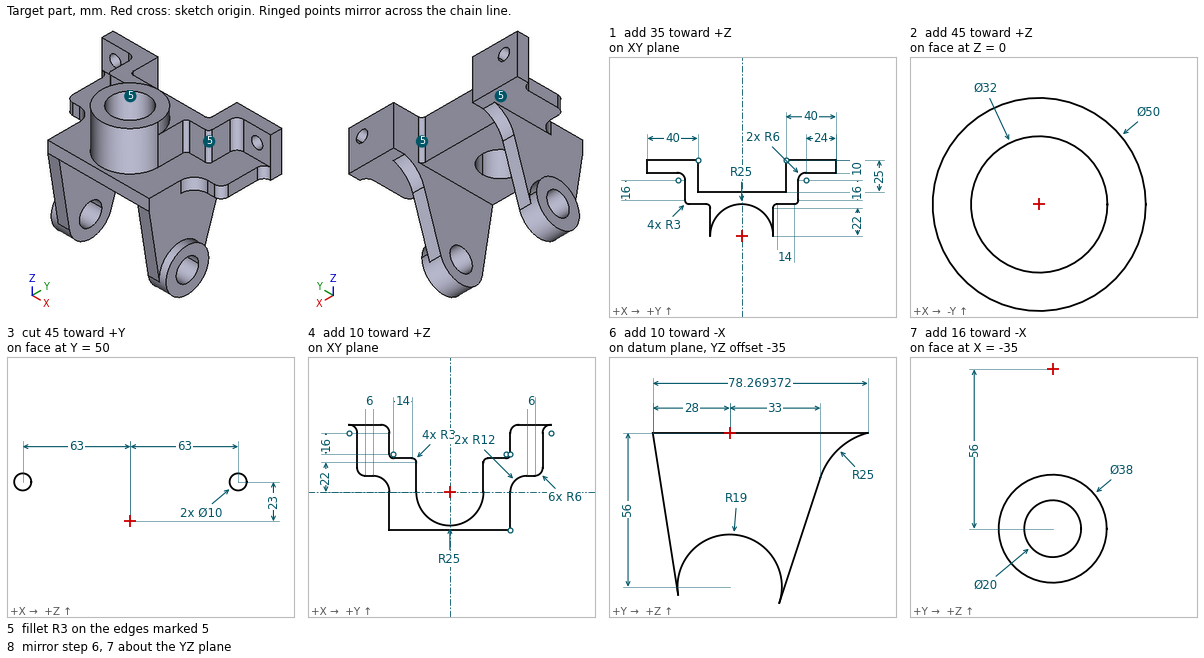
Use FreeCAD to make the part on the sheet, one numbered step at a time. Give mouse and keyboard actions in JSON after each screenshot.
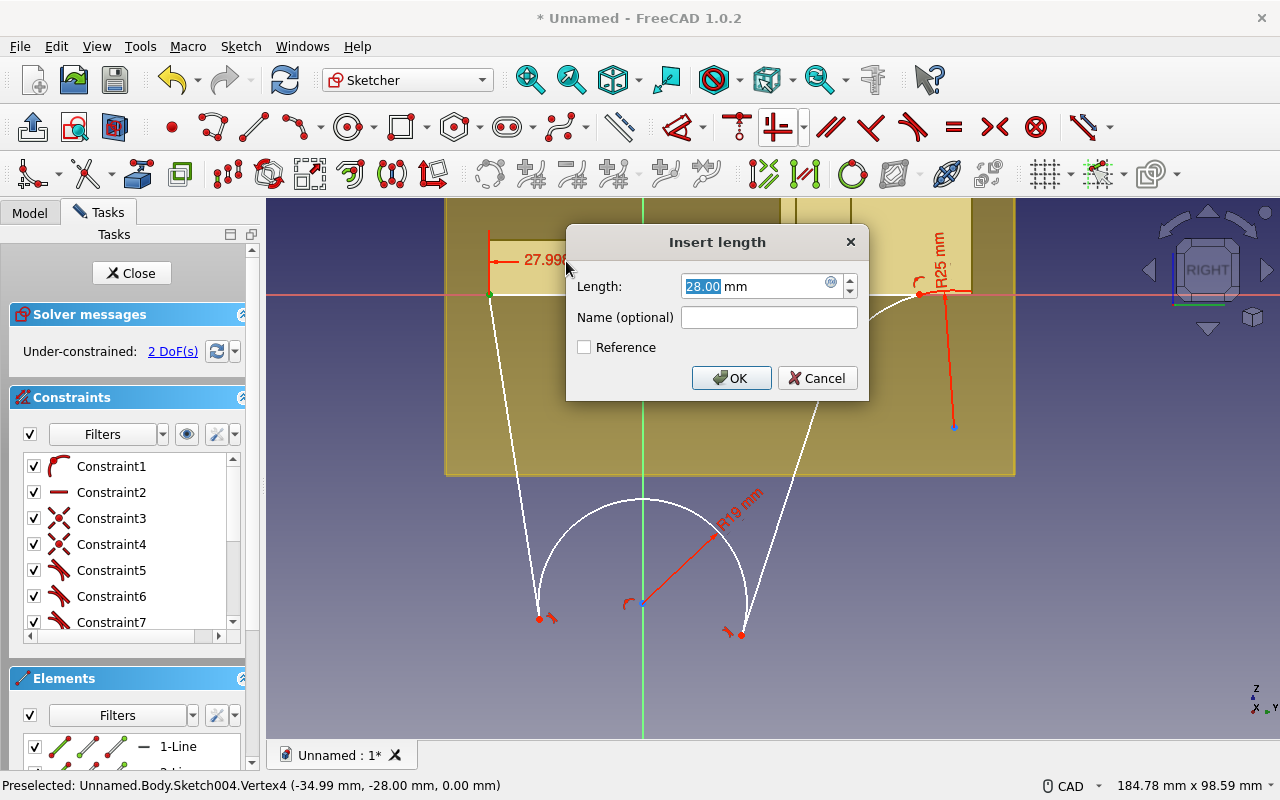
{"action": "type", "text": "28"}
{"action": "key", "text": "Return"}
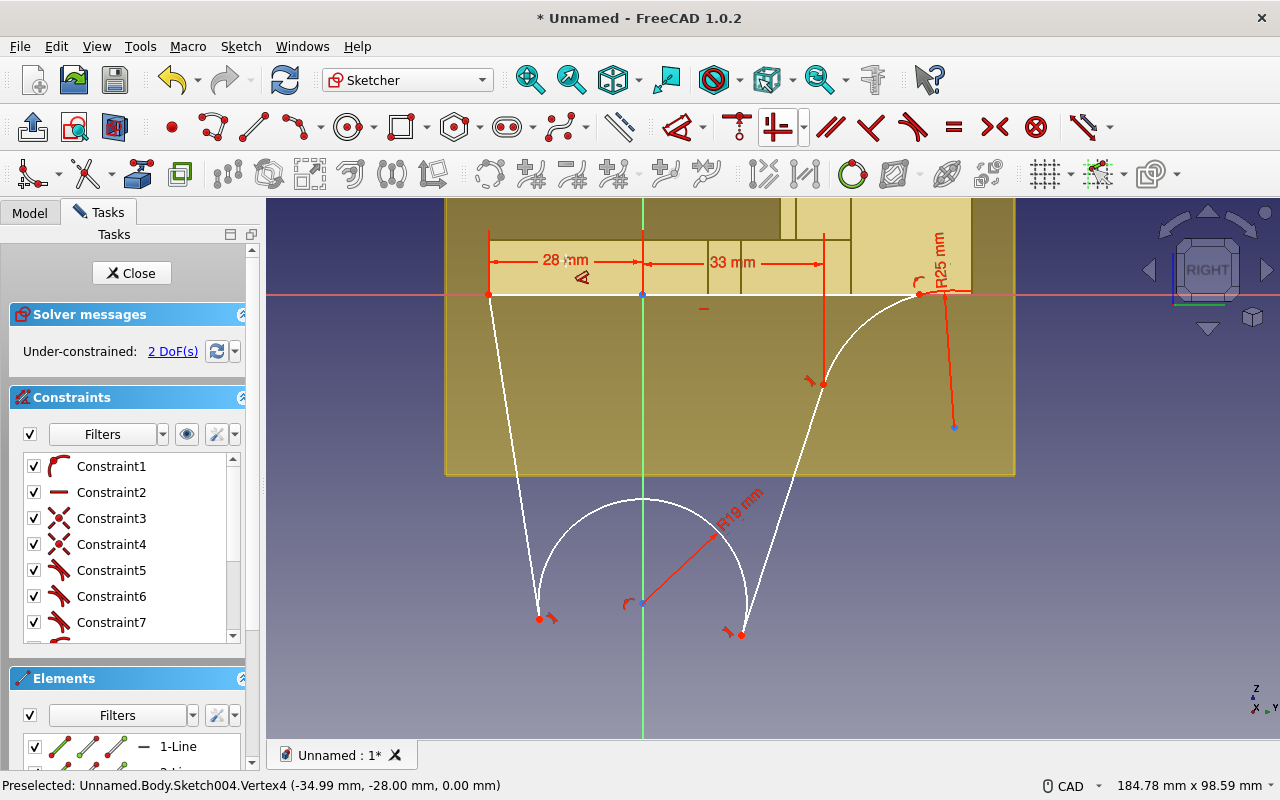
{"action": "left_click", "coordinate": [643, 603]}
{"action": "left_click", "coordinate": [609, 449]}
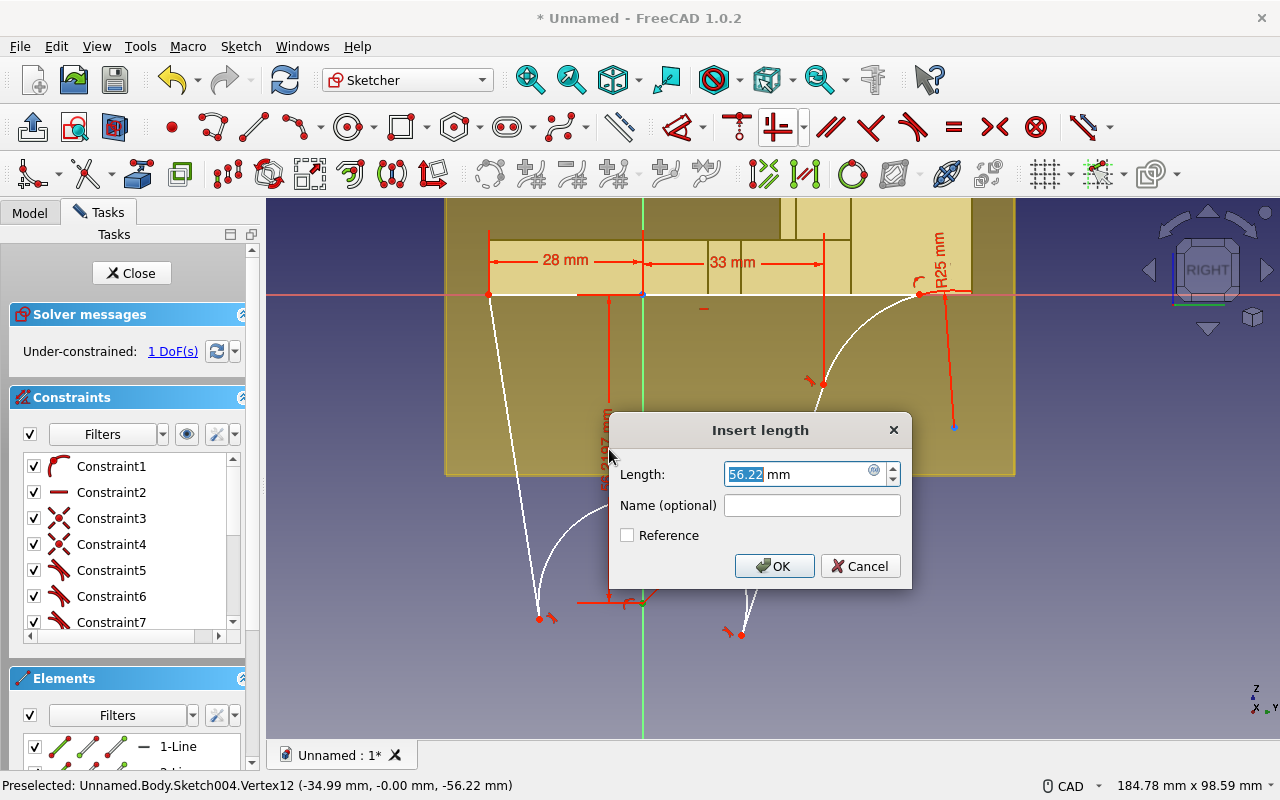
{"action": "type", "text": "56"}
{"action": "key", "text": "Return"}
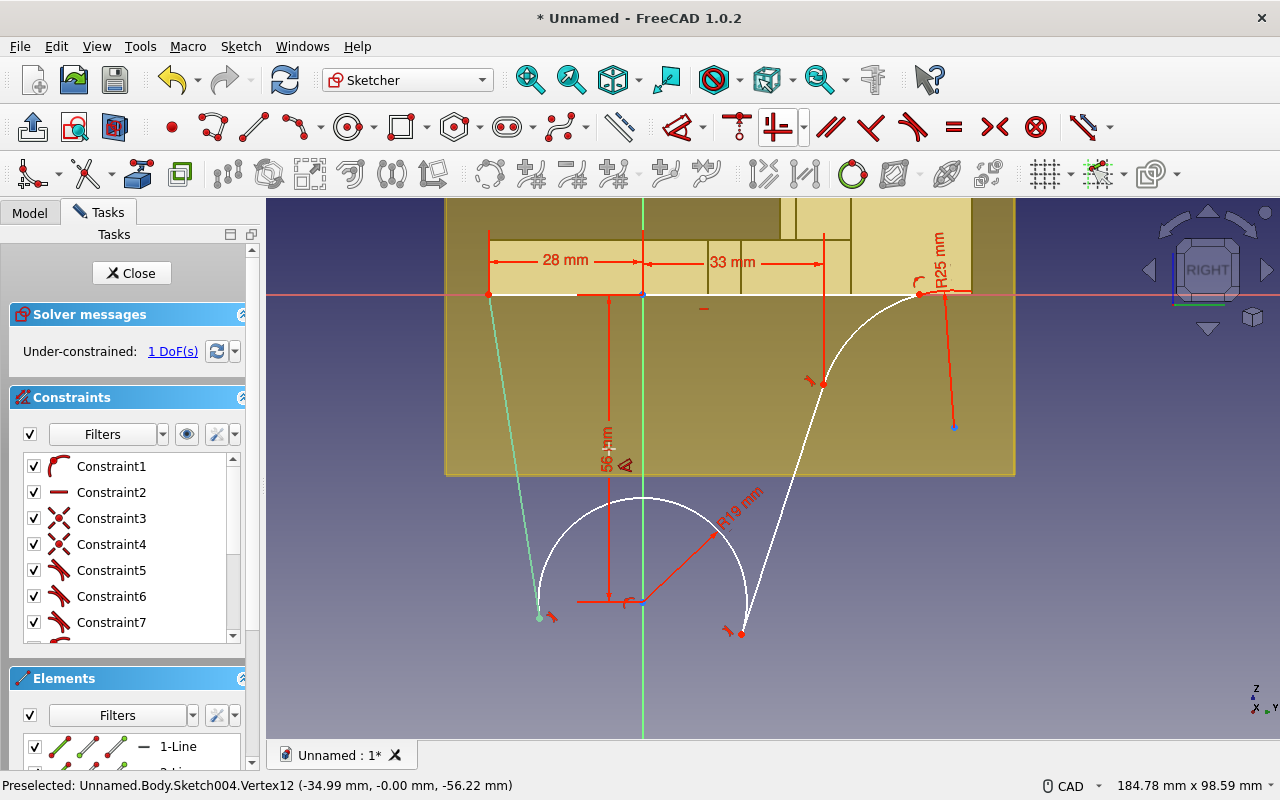
{"action": "left_click", "coordinate": [790, 295]}
{"action": "left_click", "coordinate": [855, 261]}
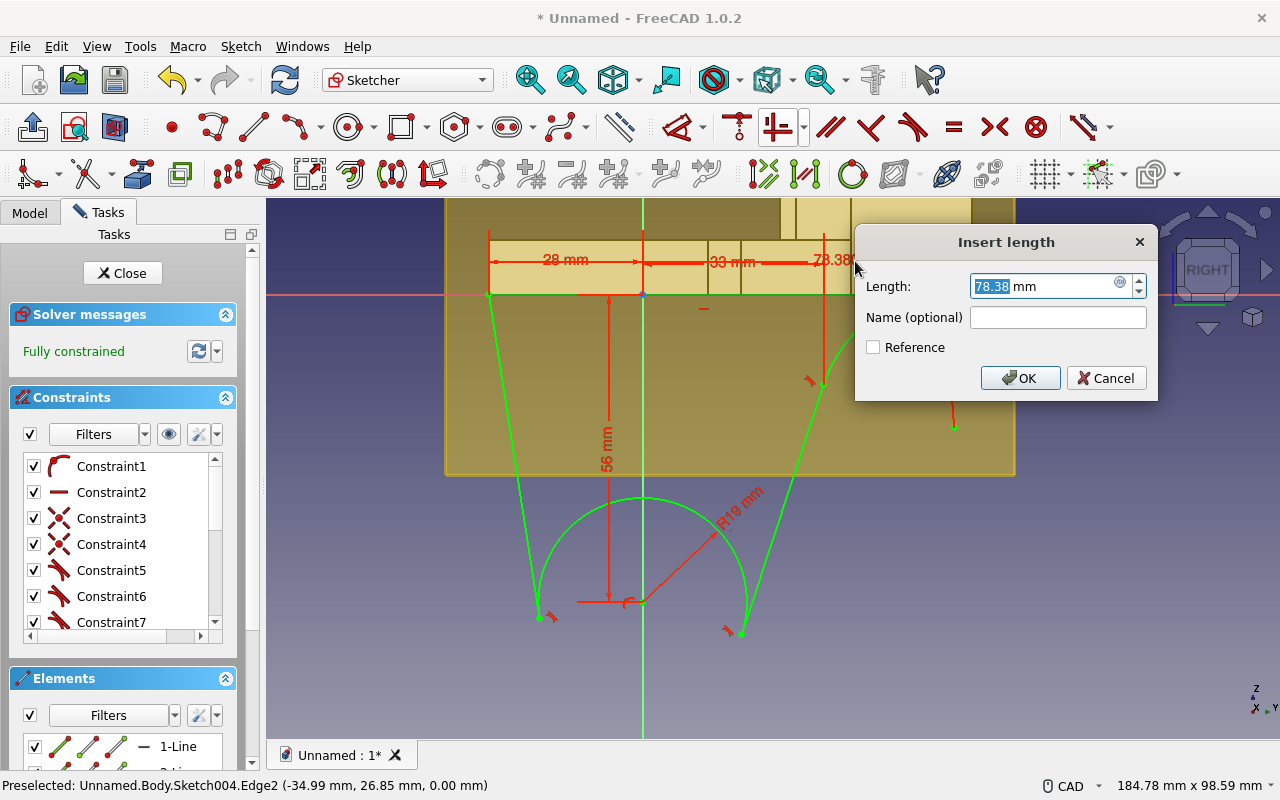
{"action": "type", "text": "78.269372"}
{"action": "key", "text": "Return"}
{"action": "key", "text": "Escape"}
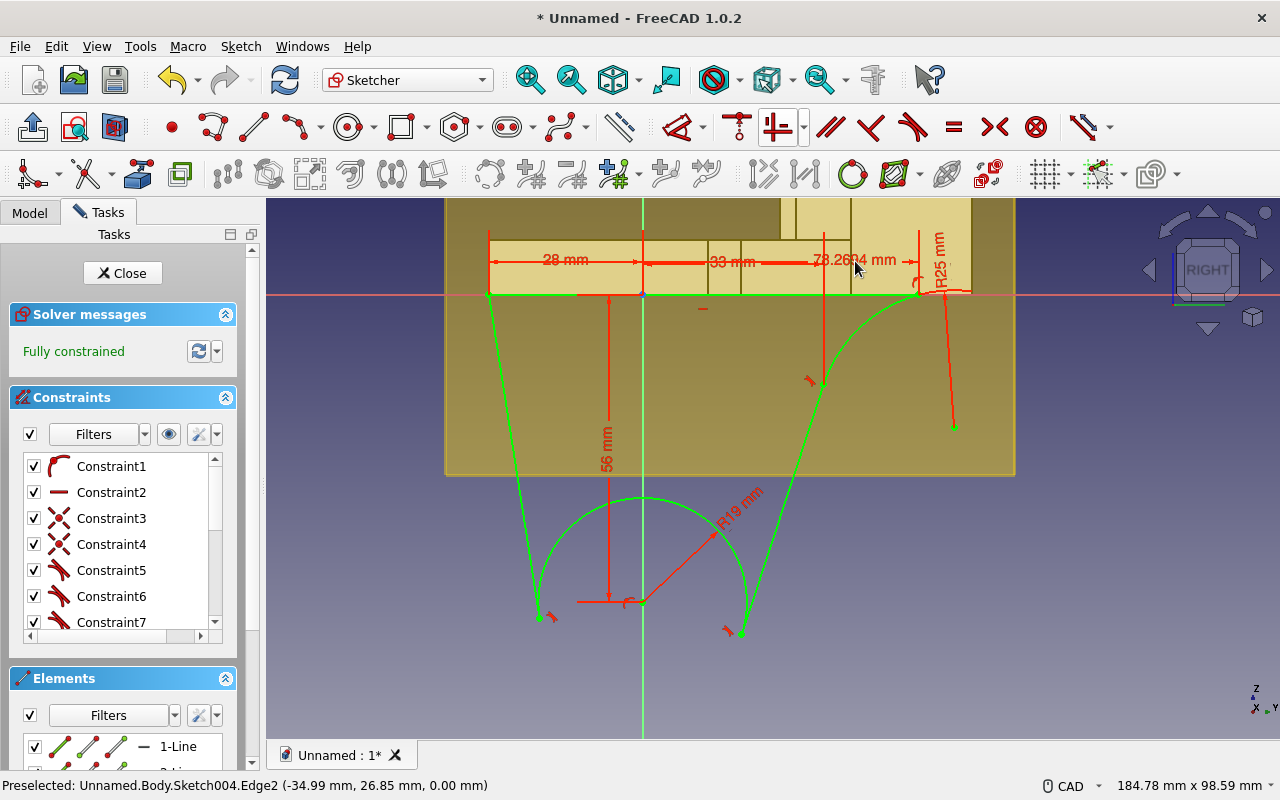
{"action": "left_click", "coordinate": [123, 273]}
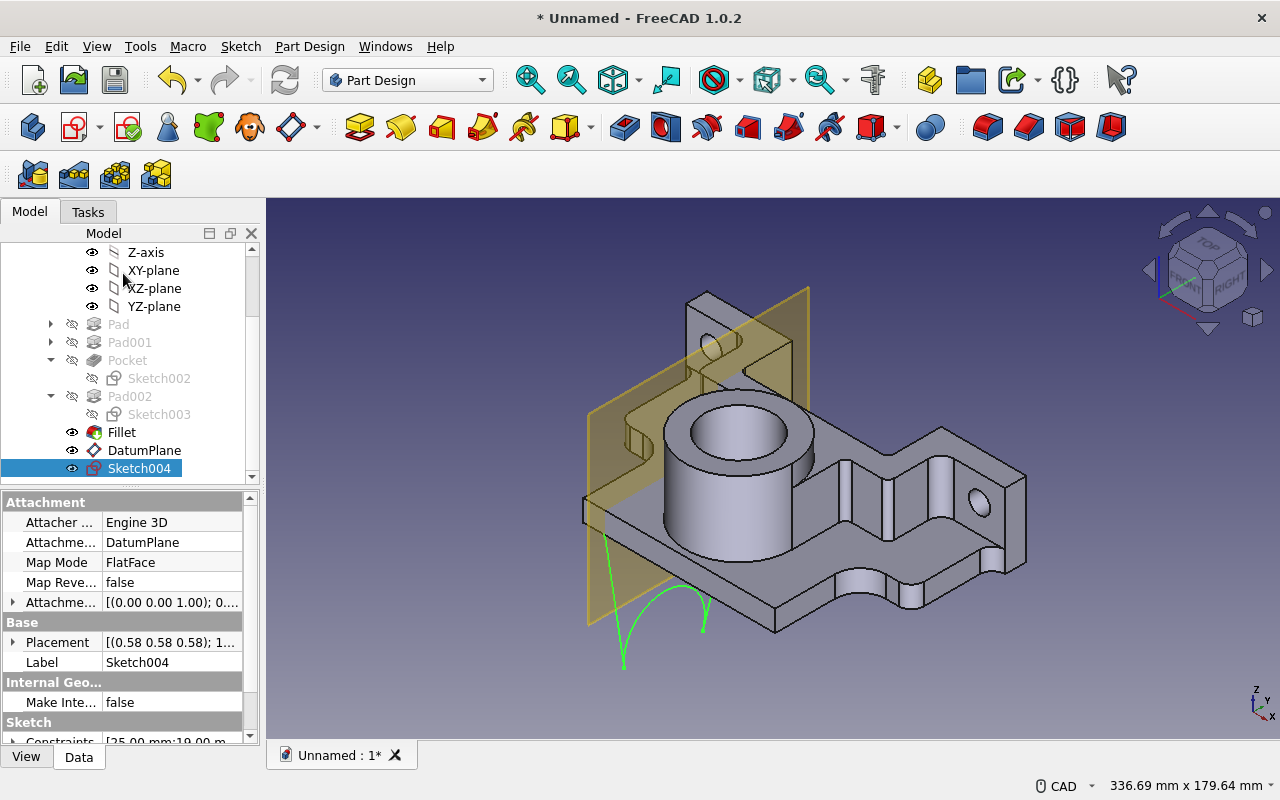
{"action": "left_click", "coordinate": [360, 128]}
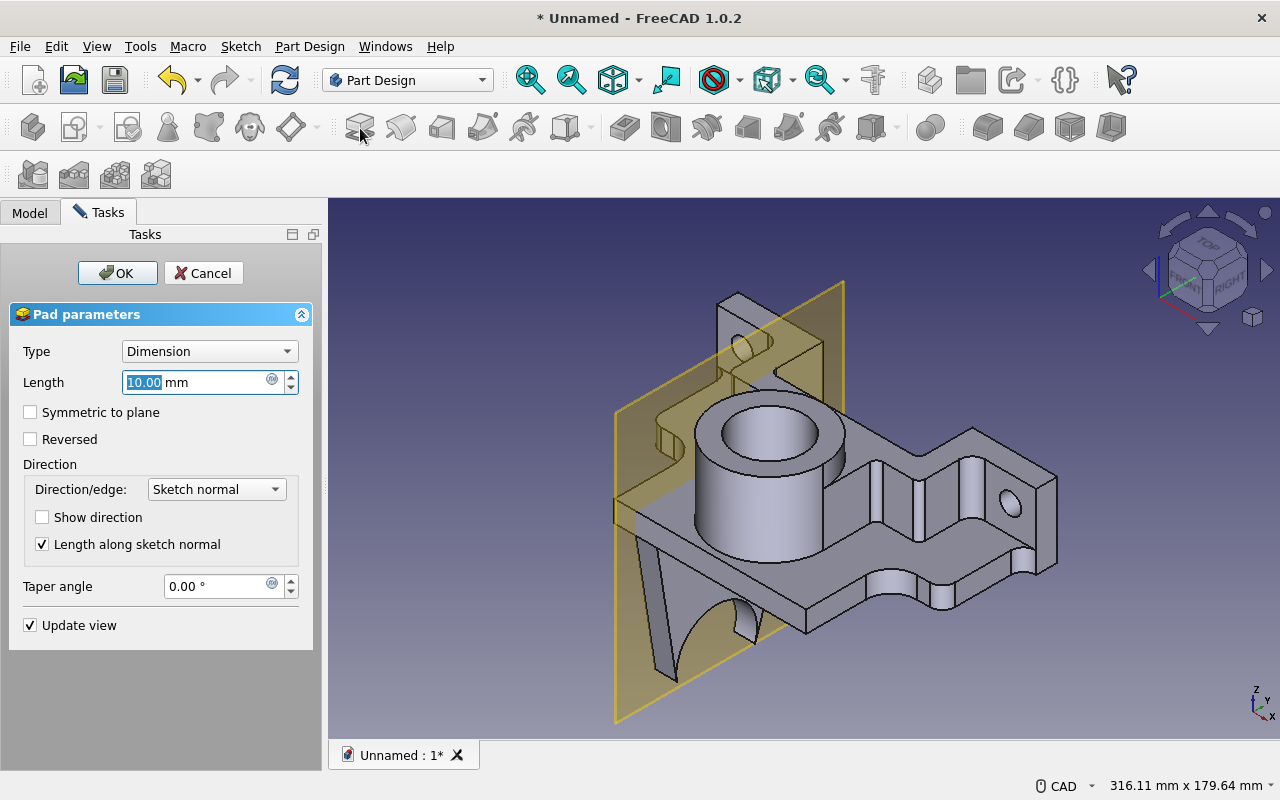
{"action": "type", "text": "10"}
{"action": "key", "text": "Tab"}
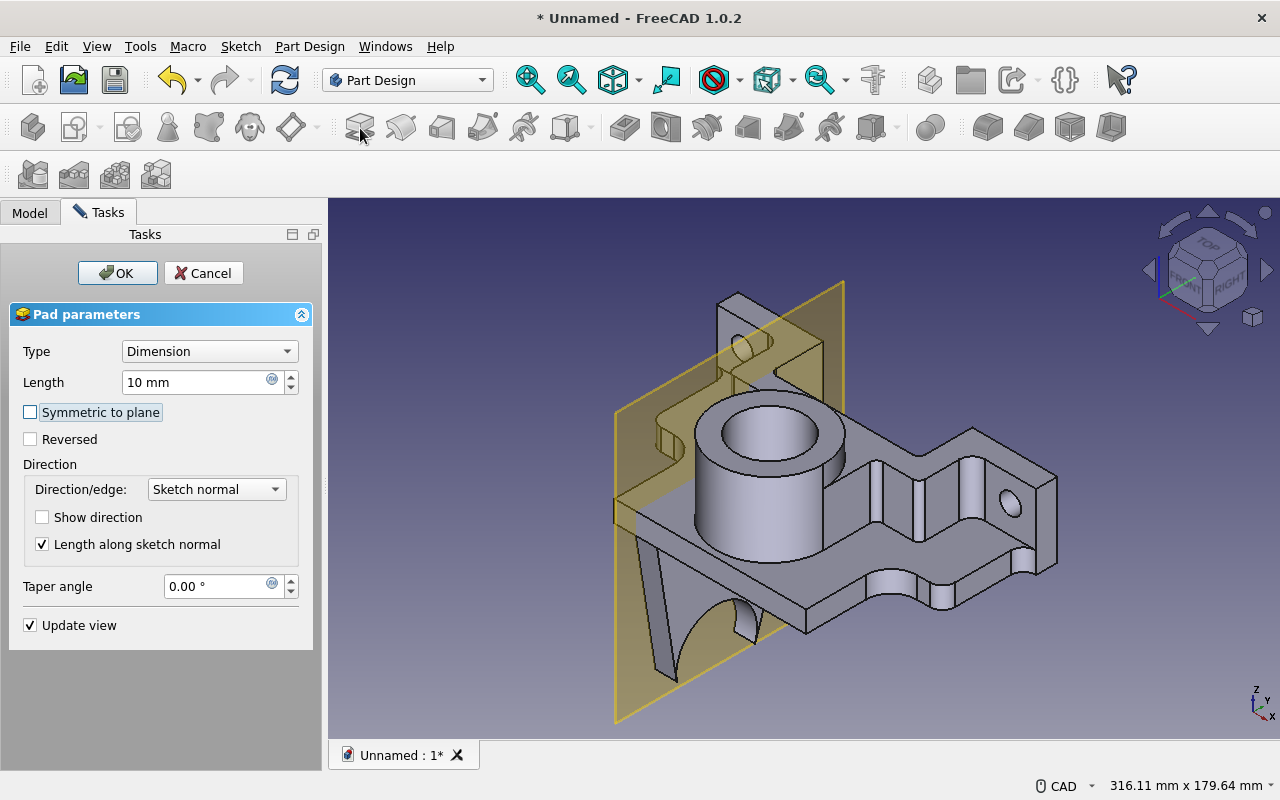
{"action": "left_click", "coordinate": [31, 439]}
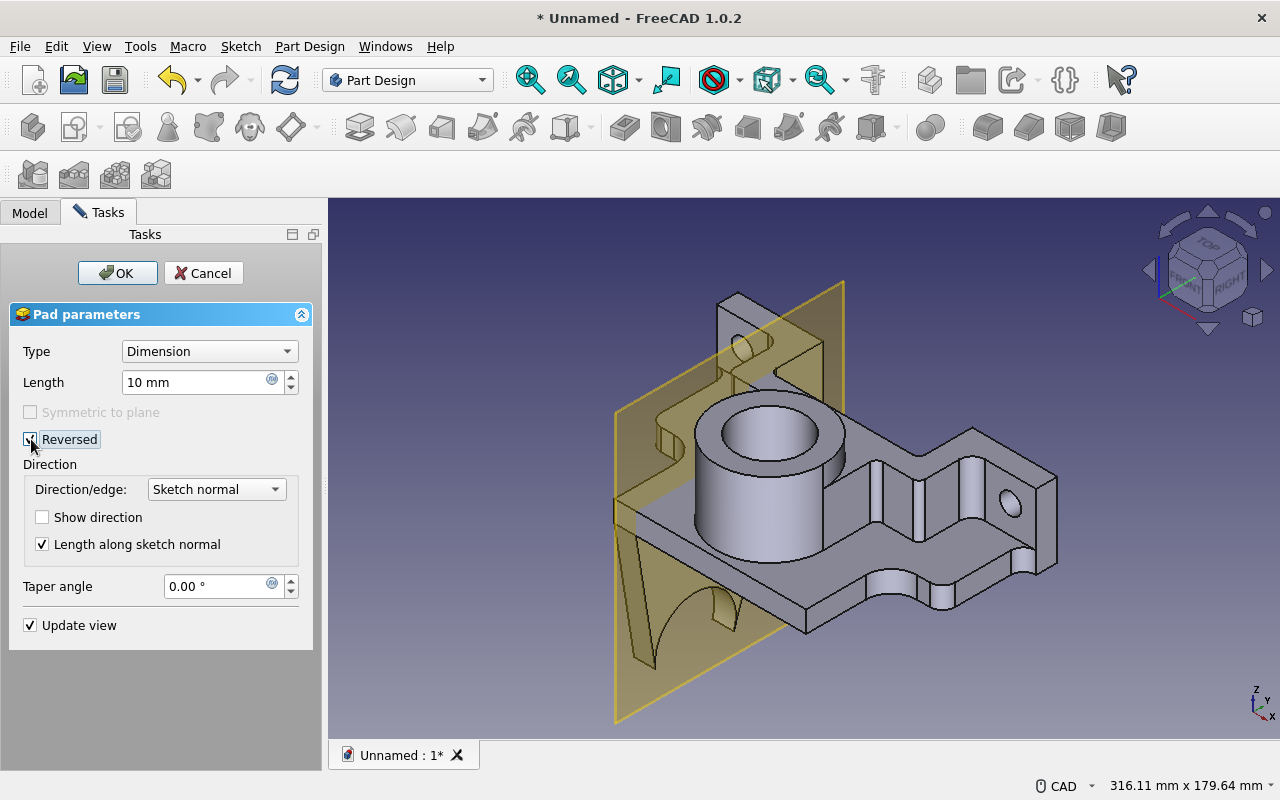
{"action": "left_click", "coordinate": [118, 273]}